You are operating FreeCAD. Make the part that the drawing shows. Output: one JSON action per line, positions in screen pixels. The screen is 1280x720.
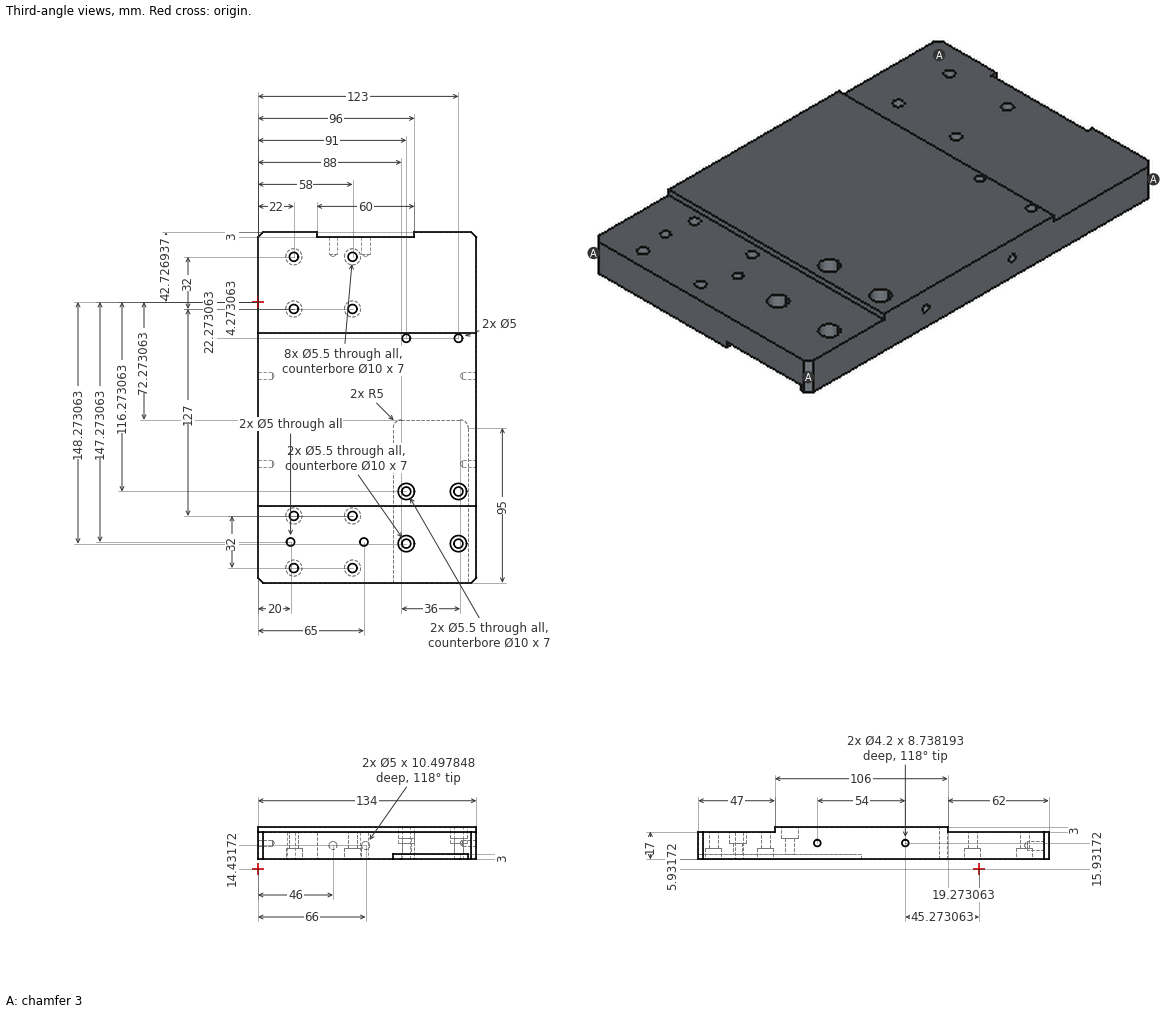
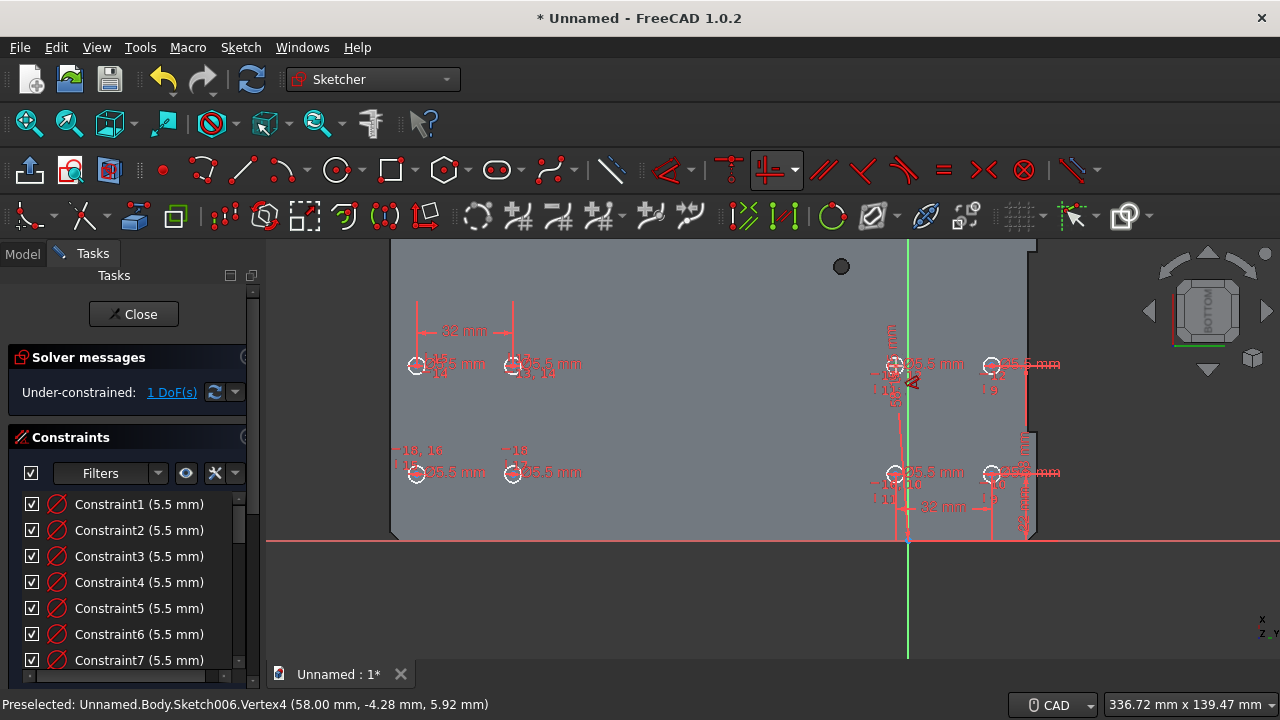
{"action": "left_click", "coordinate": [513, 366]}
{"action": "left_click", "coordinate": [704, 332]}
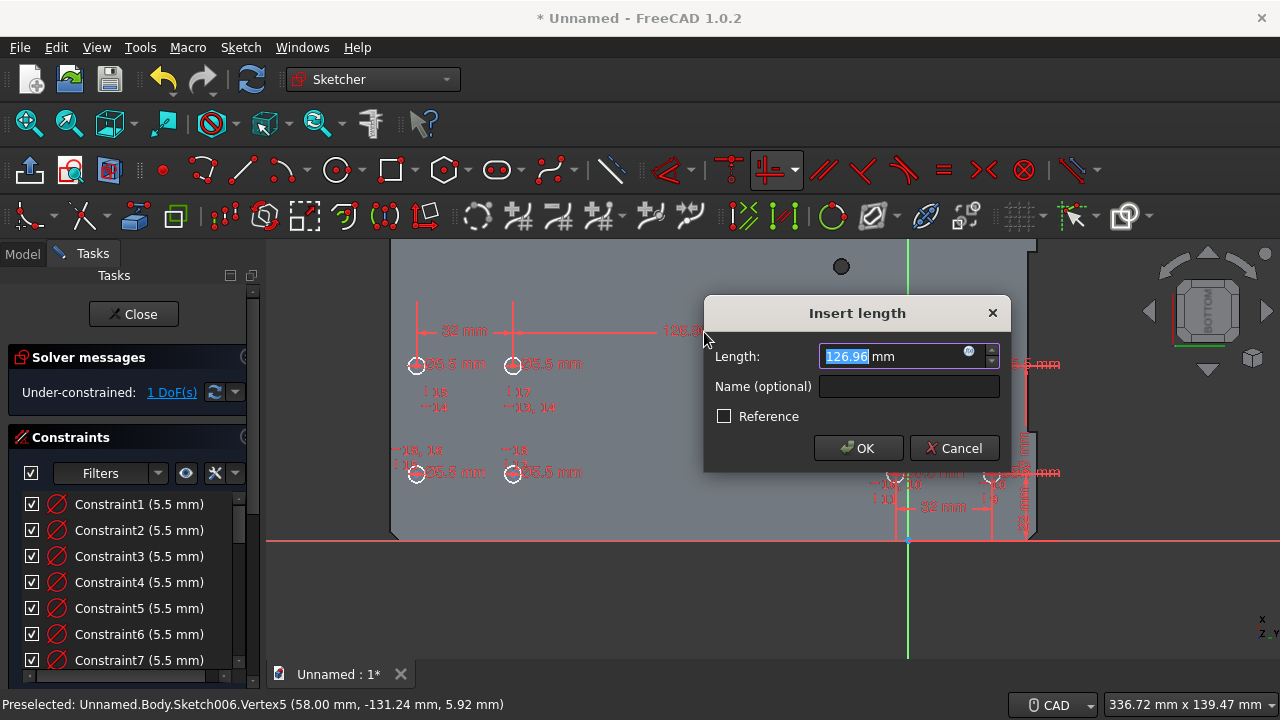
{"action": "type", "text": "127"}
{"action": "key", "text": "Return"}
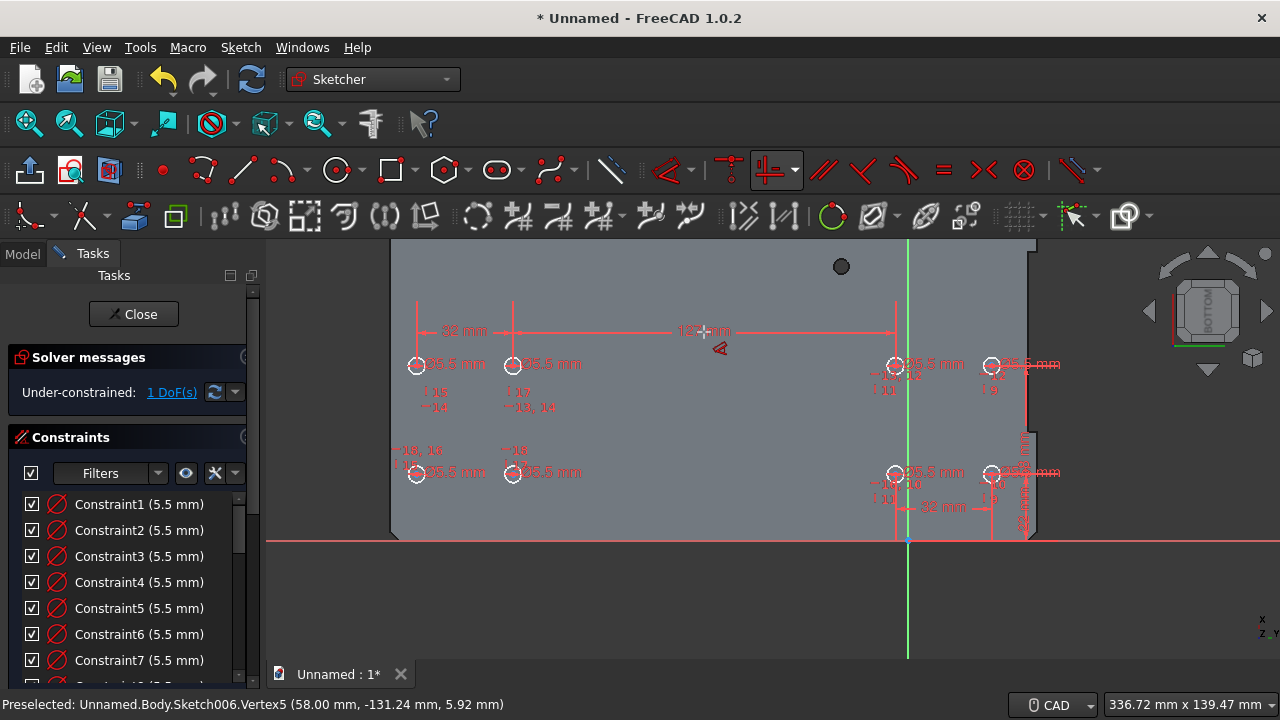
{"action": "scroll", "coordinate": [896, 474], "scroll_direction": "up", "scroll_amount": 6}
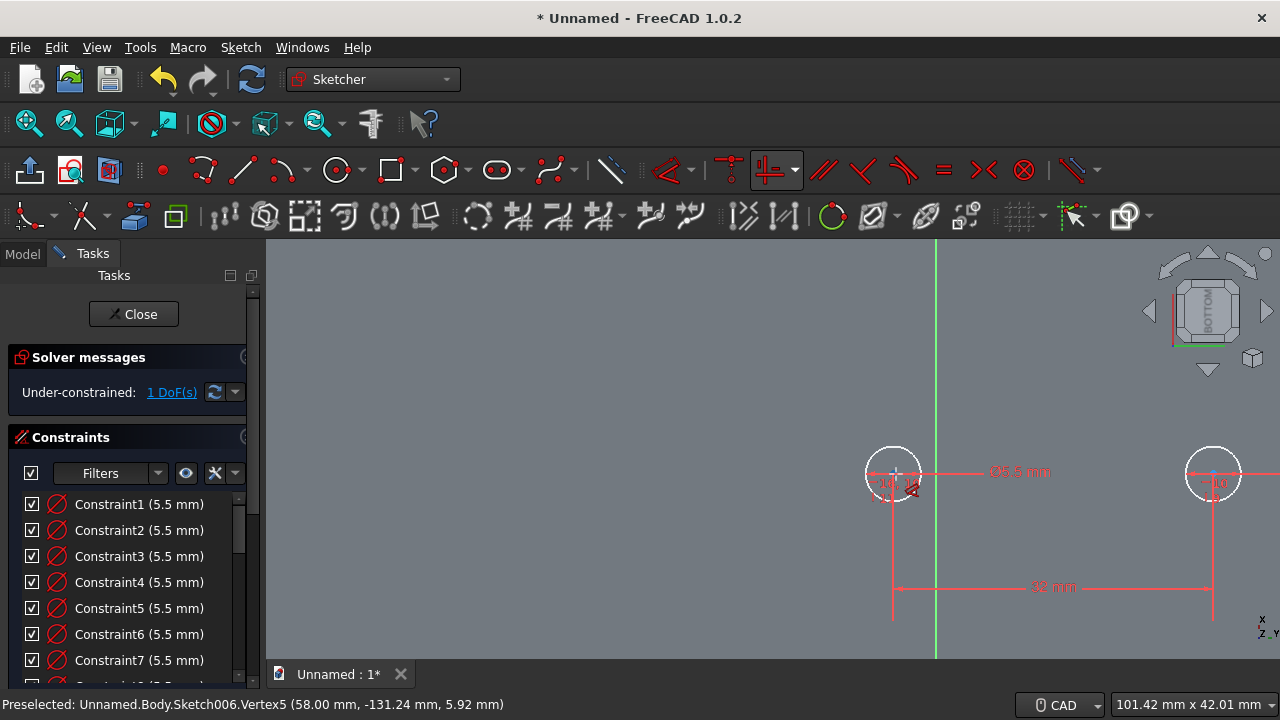
{"action": "left_click", "coordinate": [893, 474]}
{"action": "left_click", "coordinate": [915, 416]}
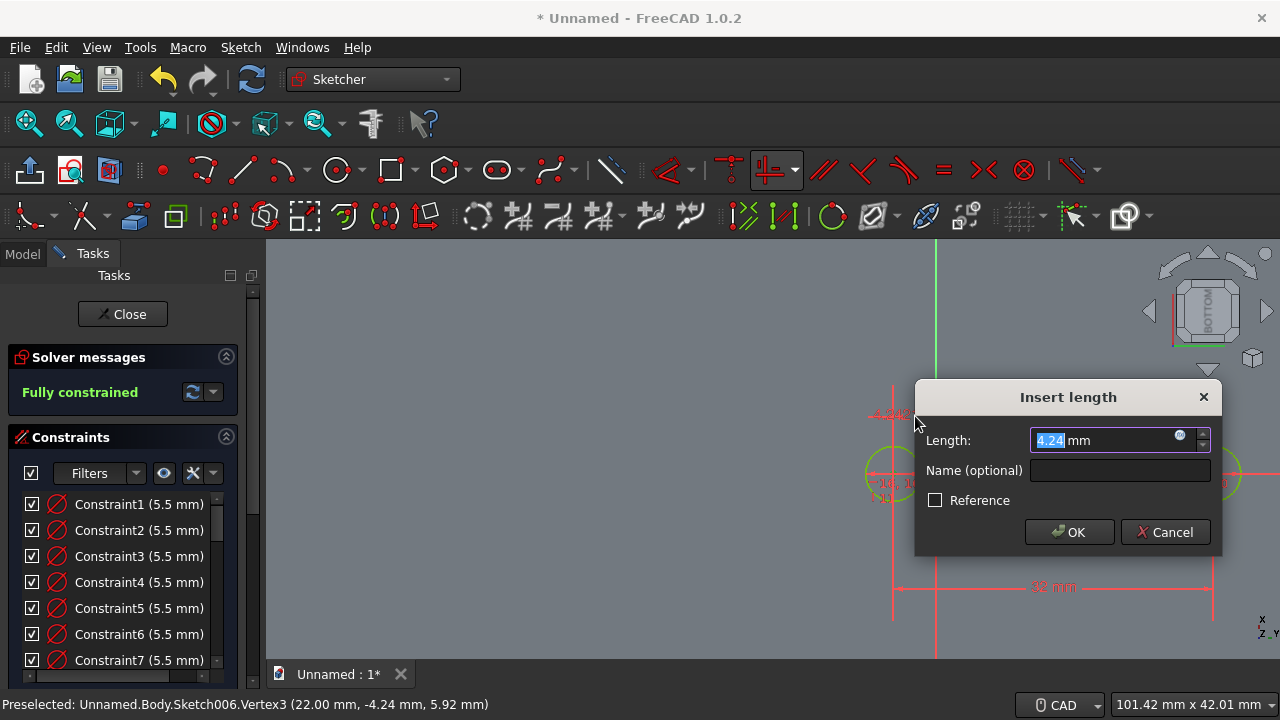
{"action": "type", "text": "4.273063"}
{"action": "key", "text": "Return"}
{"action": "key", "text": "Escape"}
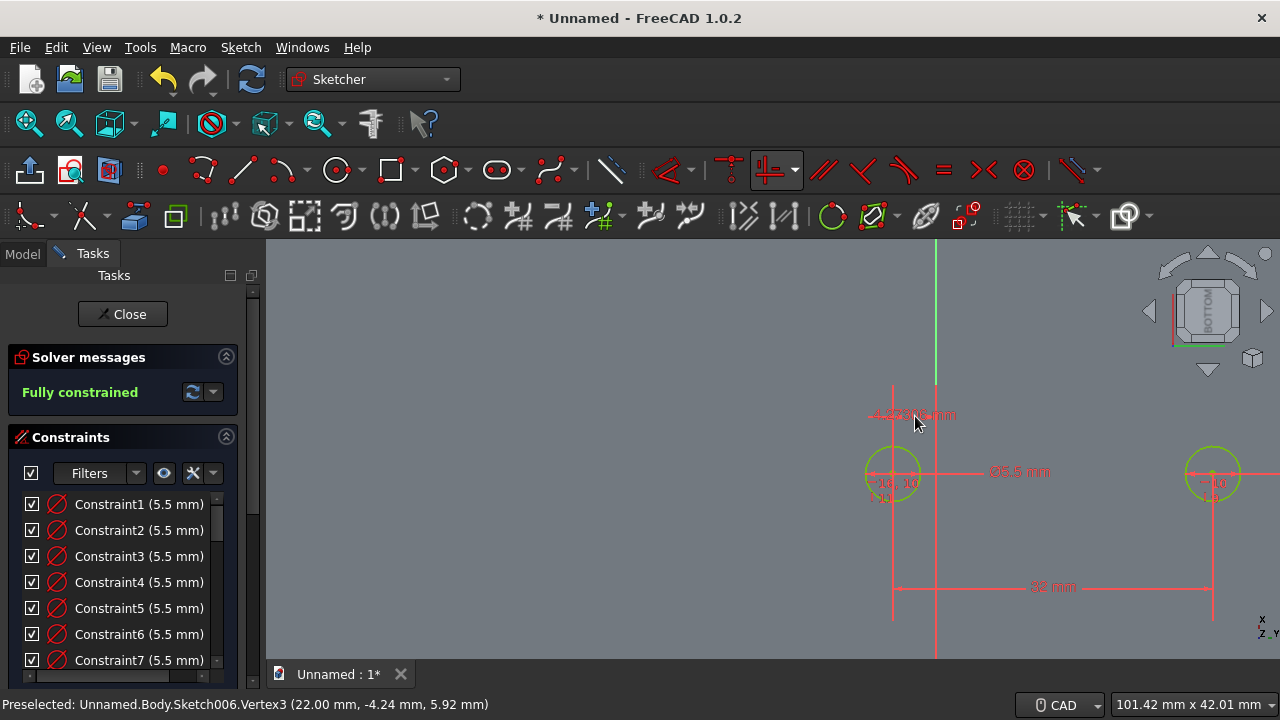
{"action": "left_click", "coordinate": [123, 314]}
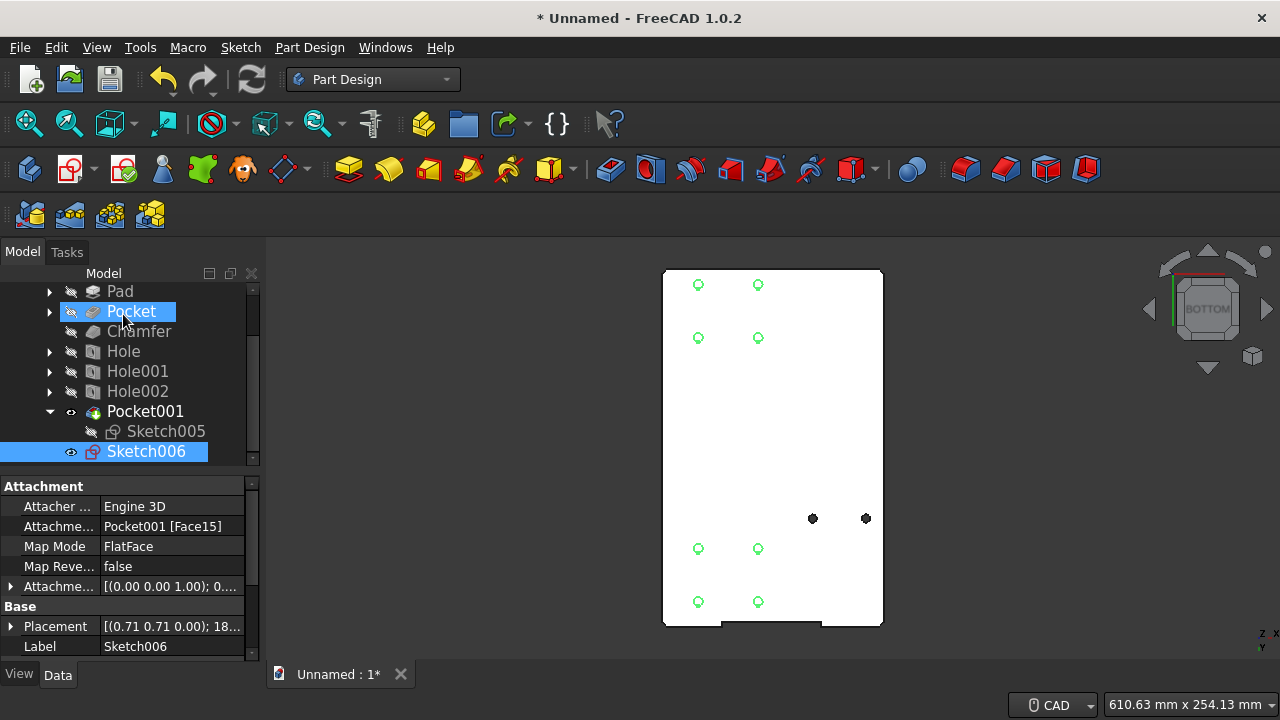
{"action": "left_click", "coordinate": [652, 170]}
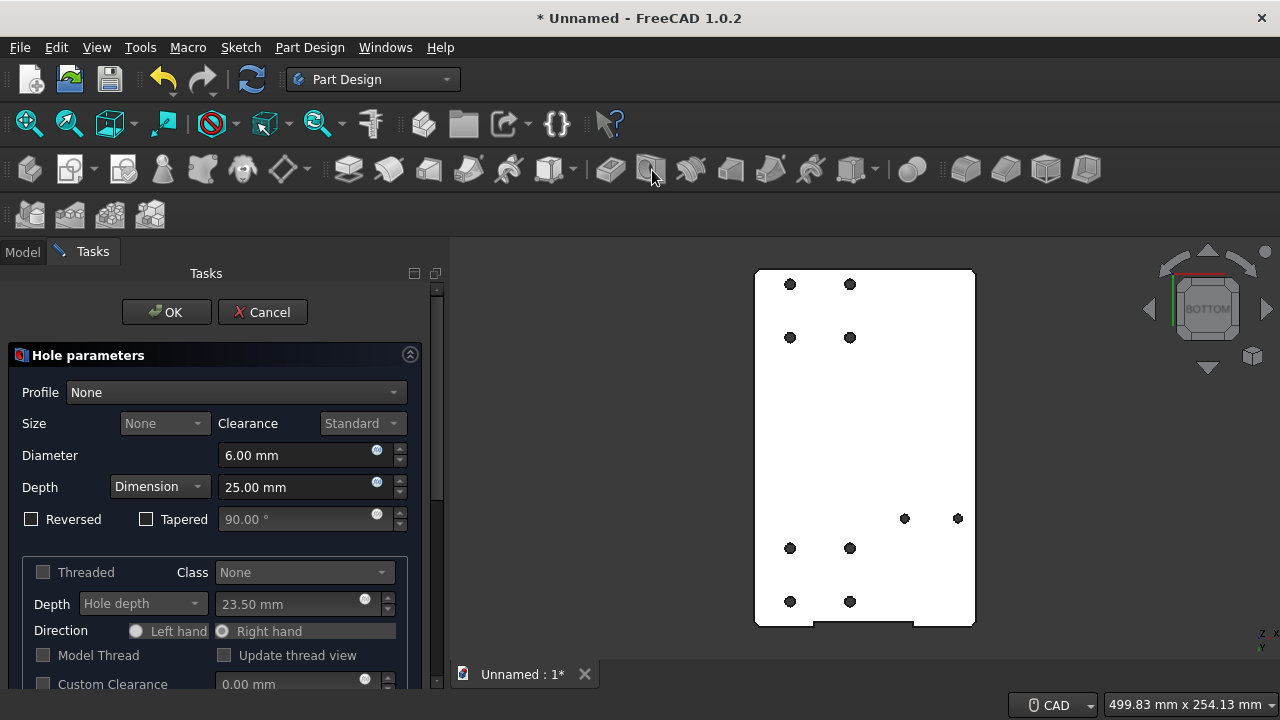
{"action": "triple_click", "coordinate": [305, 455]}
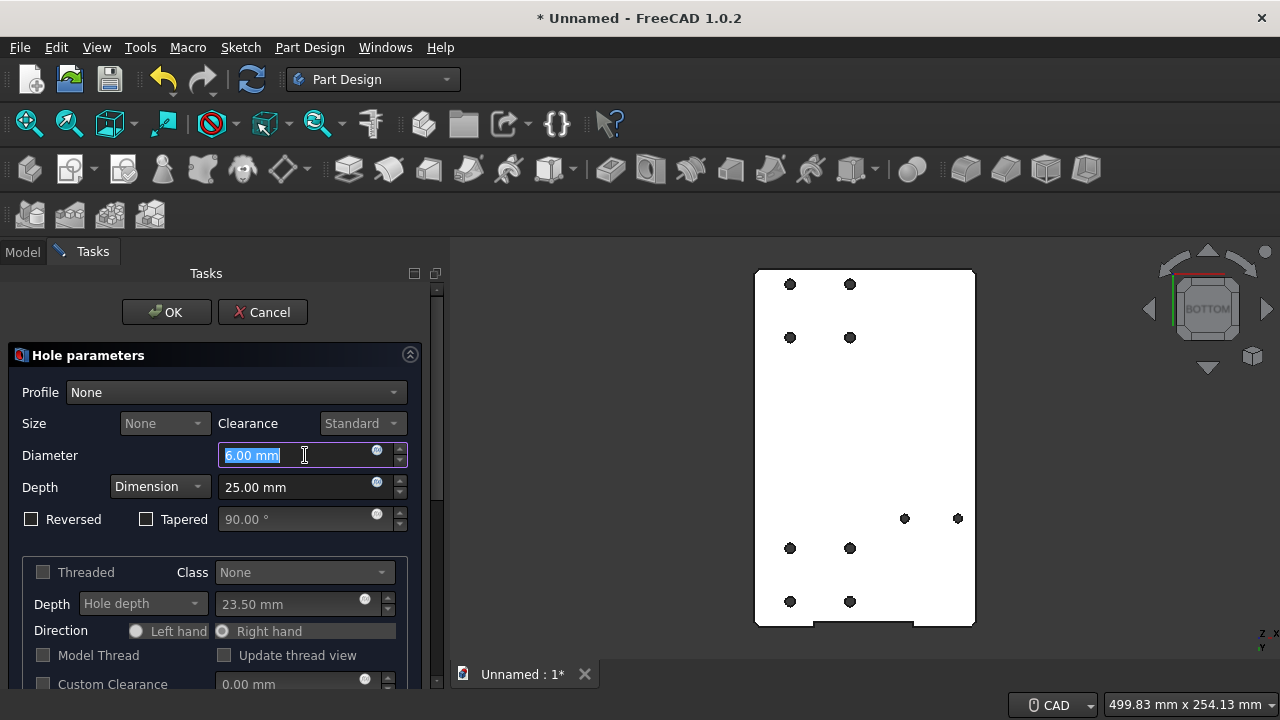
{"action": "type", "text": "5.5"}
{"action": "key", "text": "Tab"}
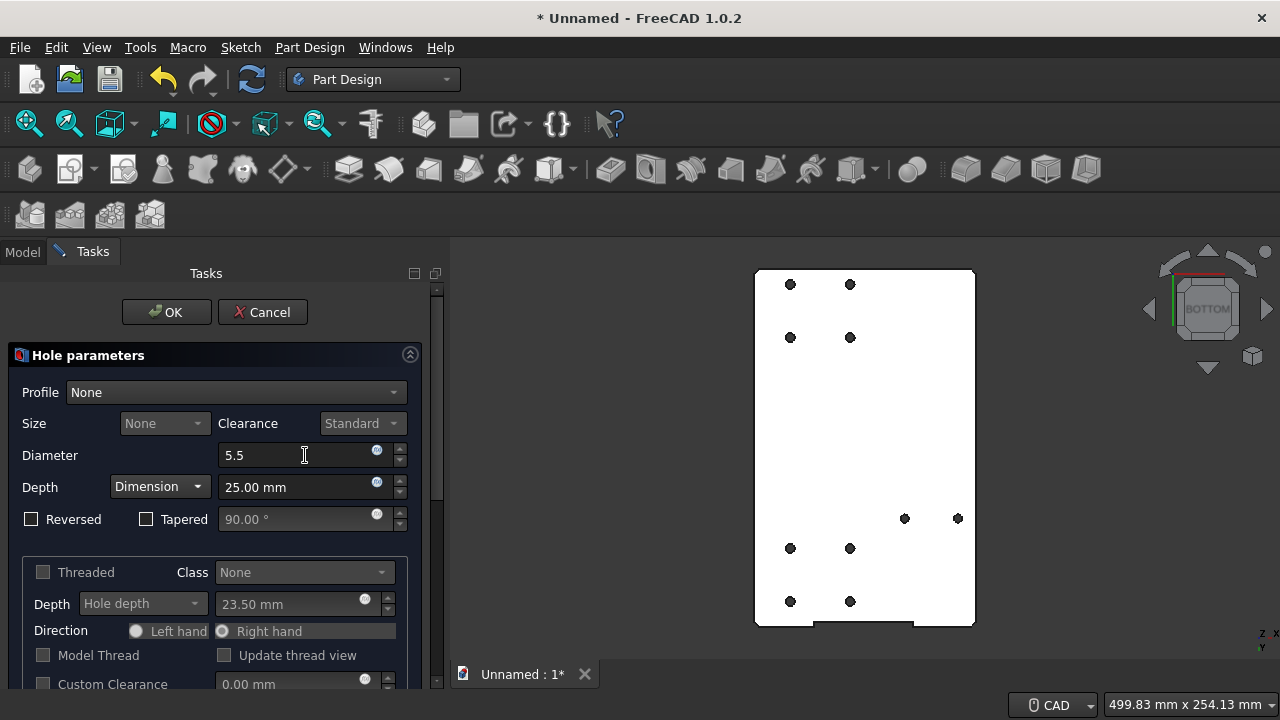
{"action": "left_click", "coordinate": [161, 486]}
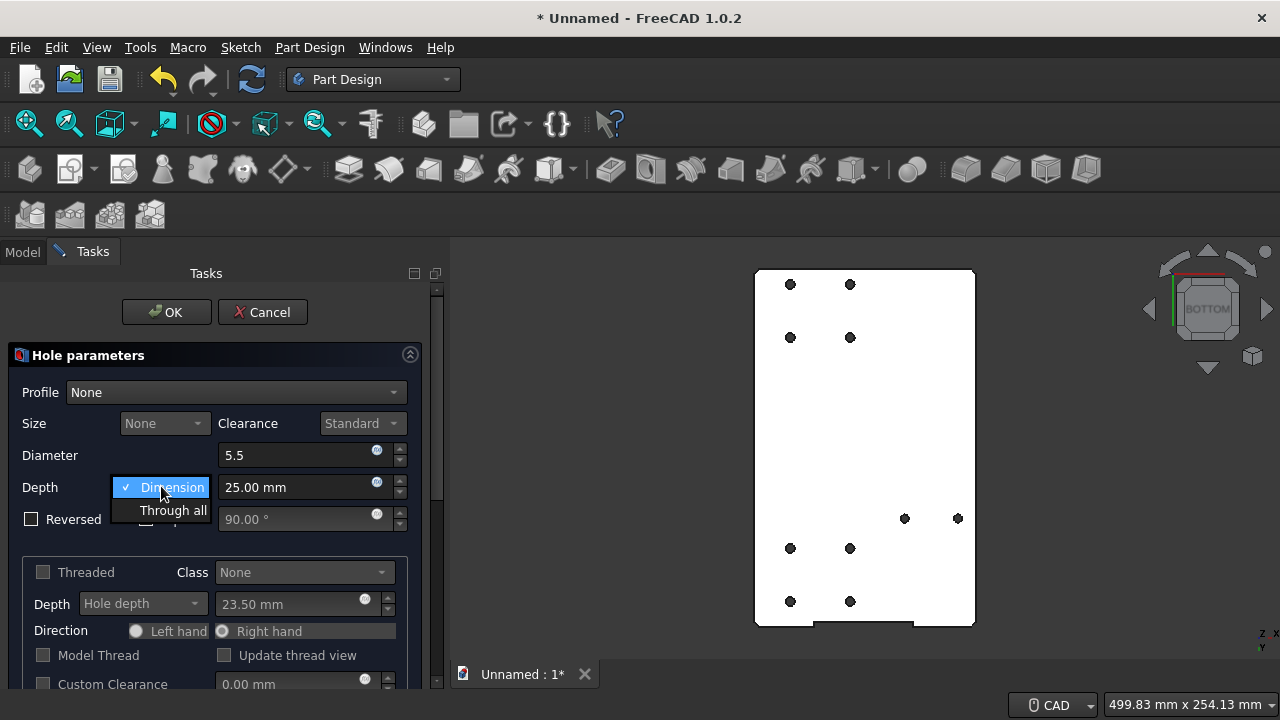
{"action": "left_click", "coordinate": [160, 510]}